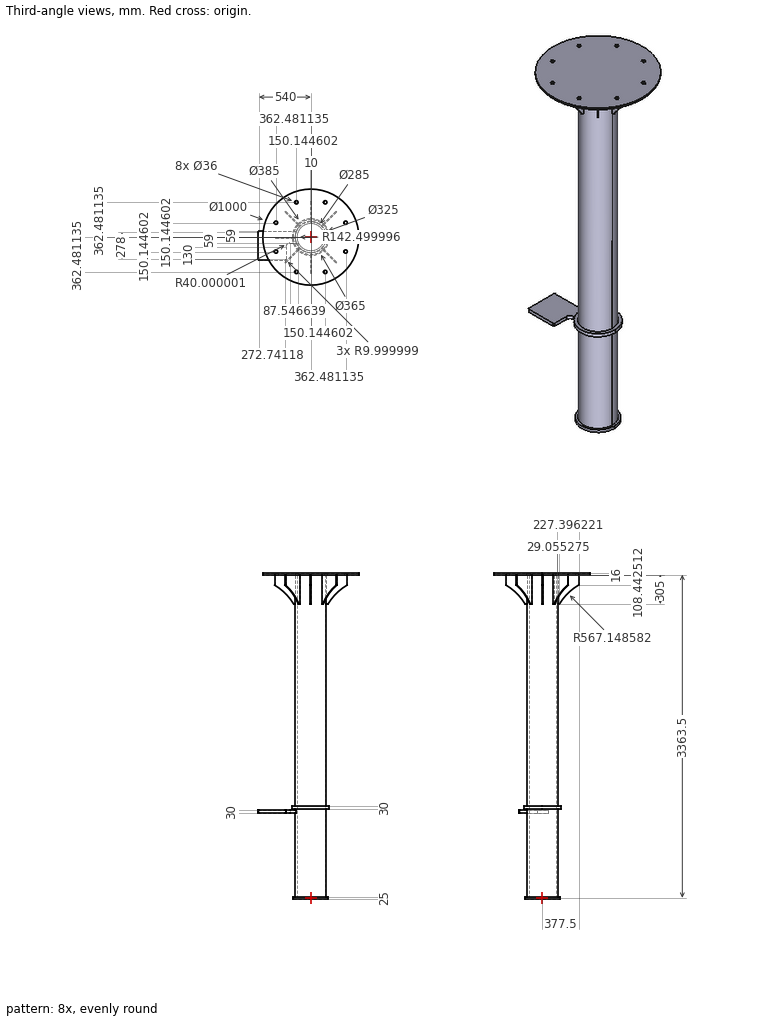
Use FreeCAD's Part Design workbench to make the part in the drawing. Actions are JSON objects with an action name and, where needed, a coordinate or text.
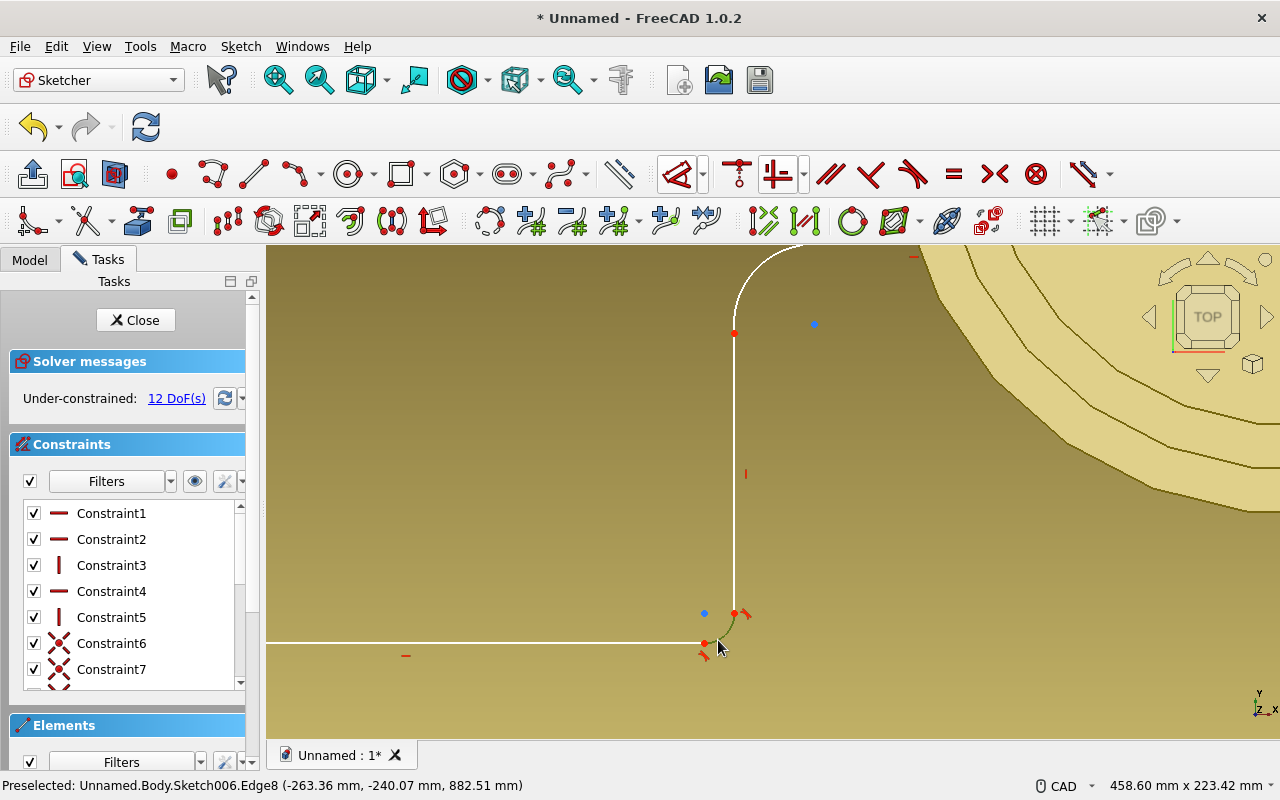
{"action": "scroll", "coordinate": [718, 640], "scroll_direction": "down", "scroll_amount": 4}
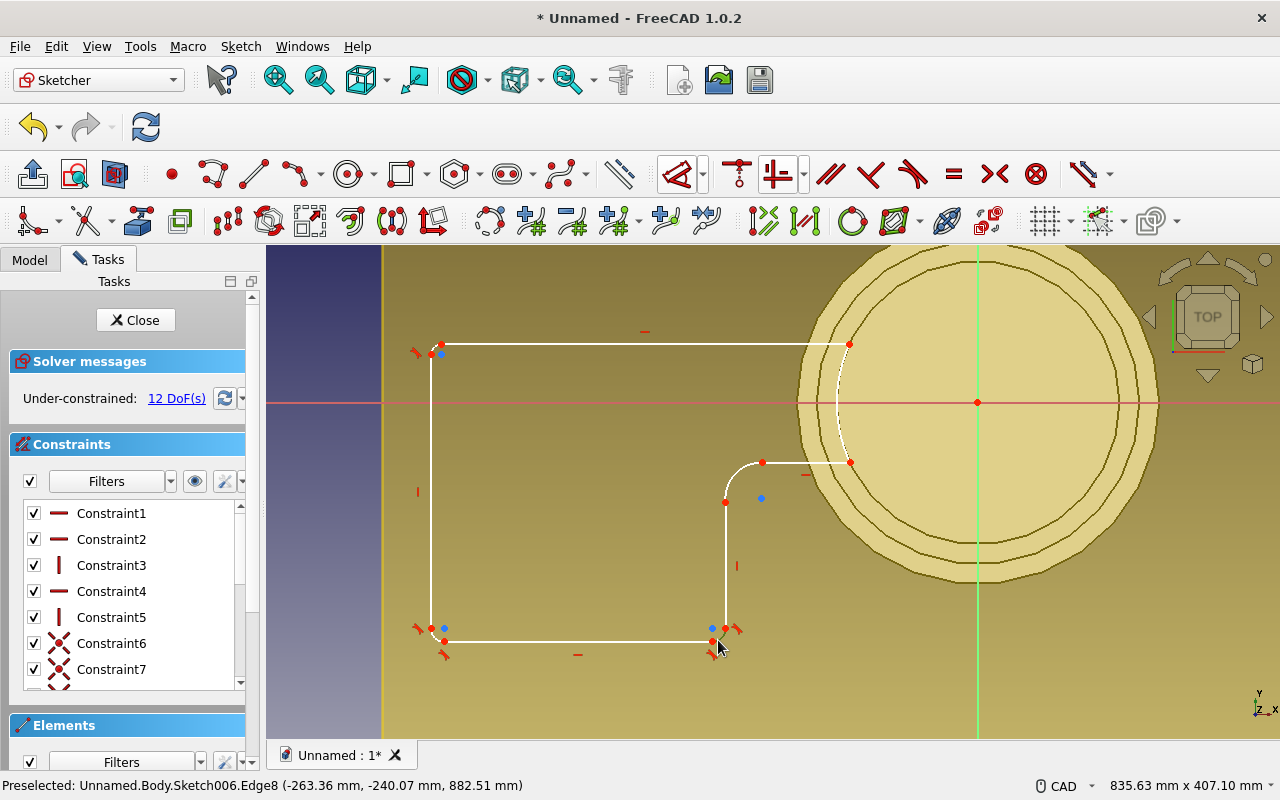
{"action": "scroll", "coordinate": [433, 635], "scroll_direction": "up", "scroll_amount": 5}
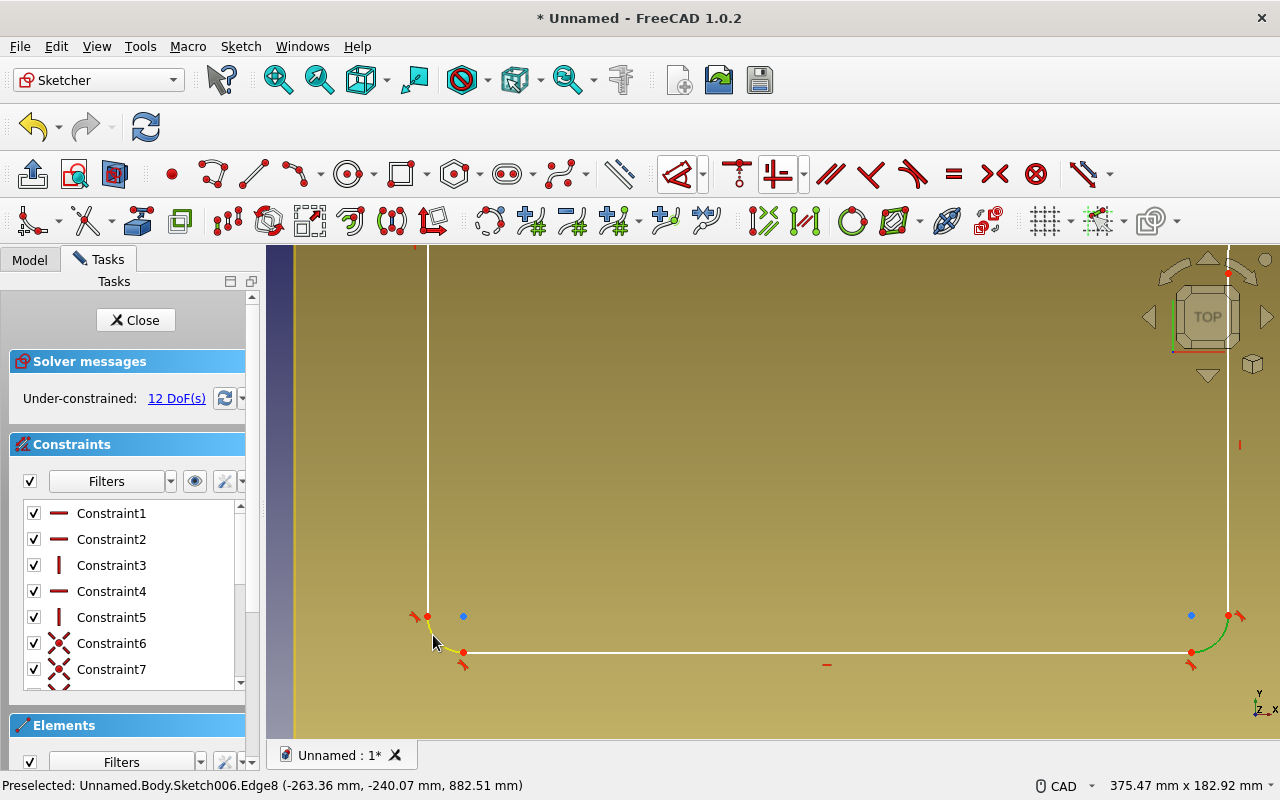
{"action": "left_click", "coordinate": [432, 633]}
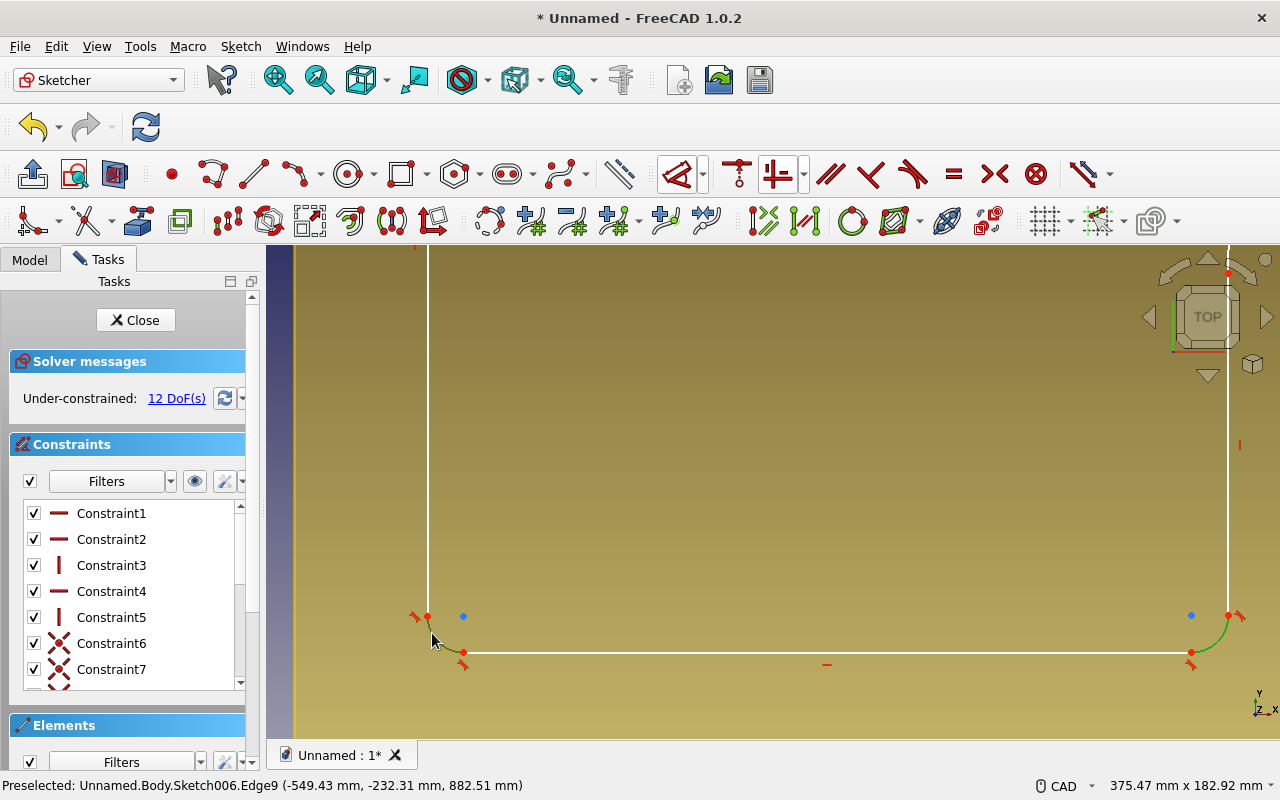
{"action": "scroll", "coordinate": [433, 635], "scroll_direction": "down", "scroll_amount": 5}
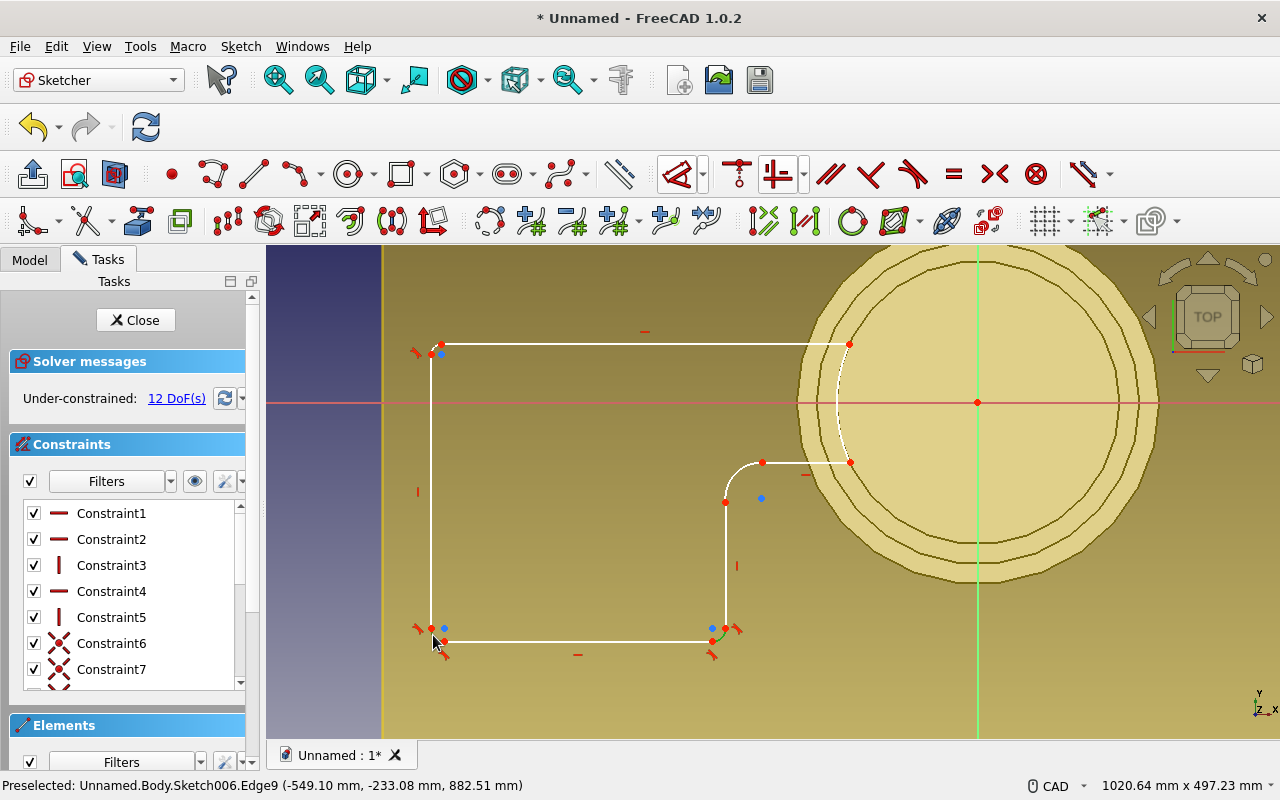
{"action": "scroll", "coordinate": [437, 345], "scroll_direction": "up", "scroll_amount": 6}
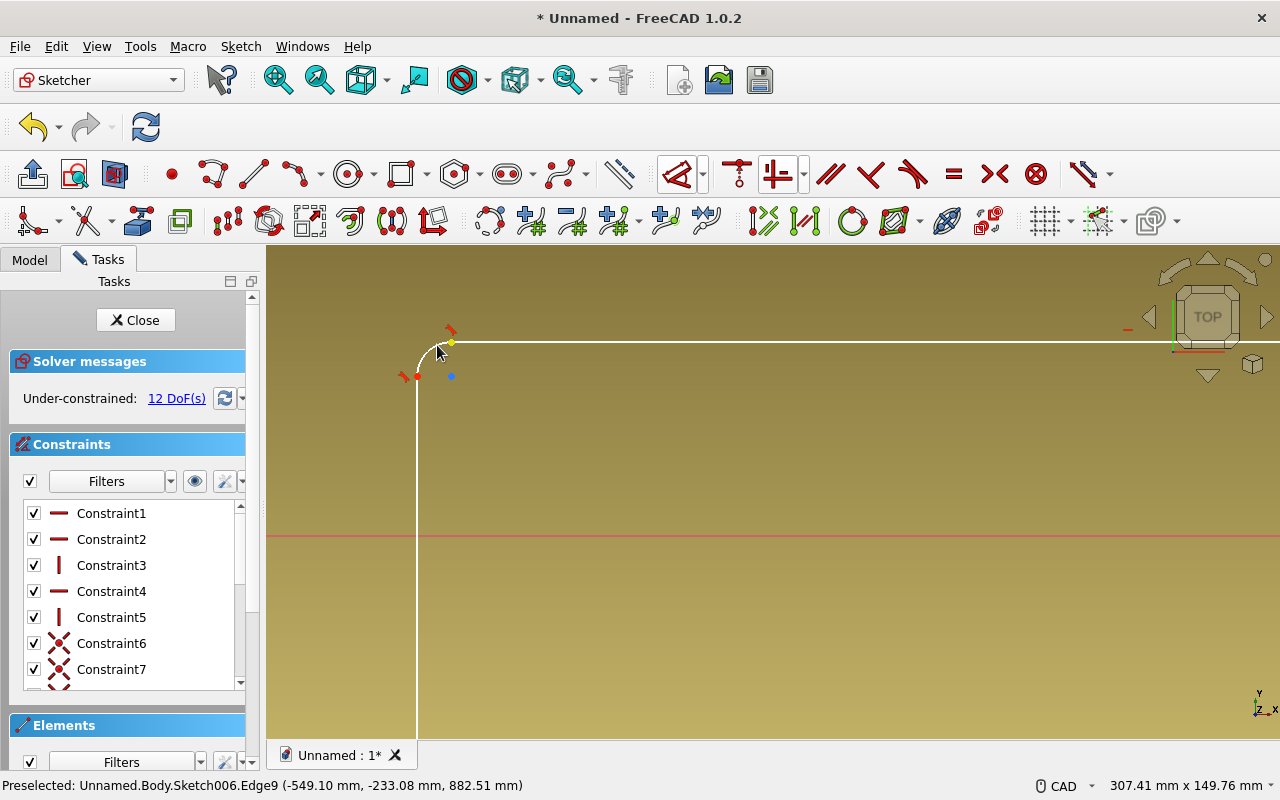
{"action": "left_click", "coordinate": [436, 346]}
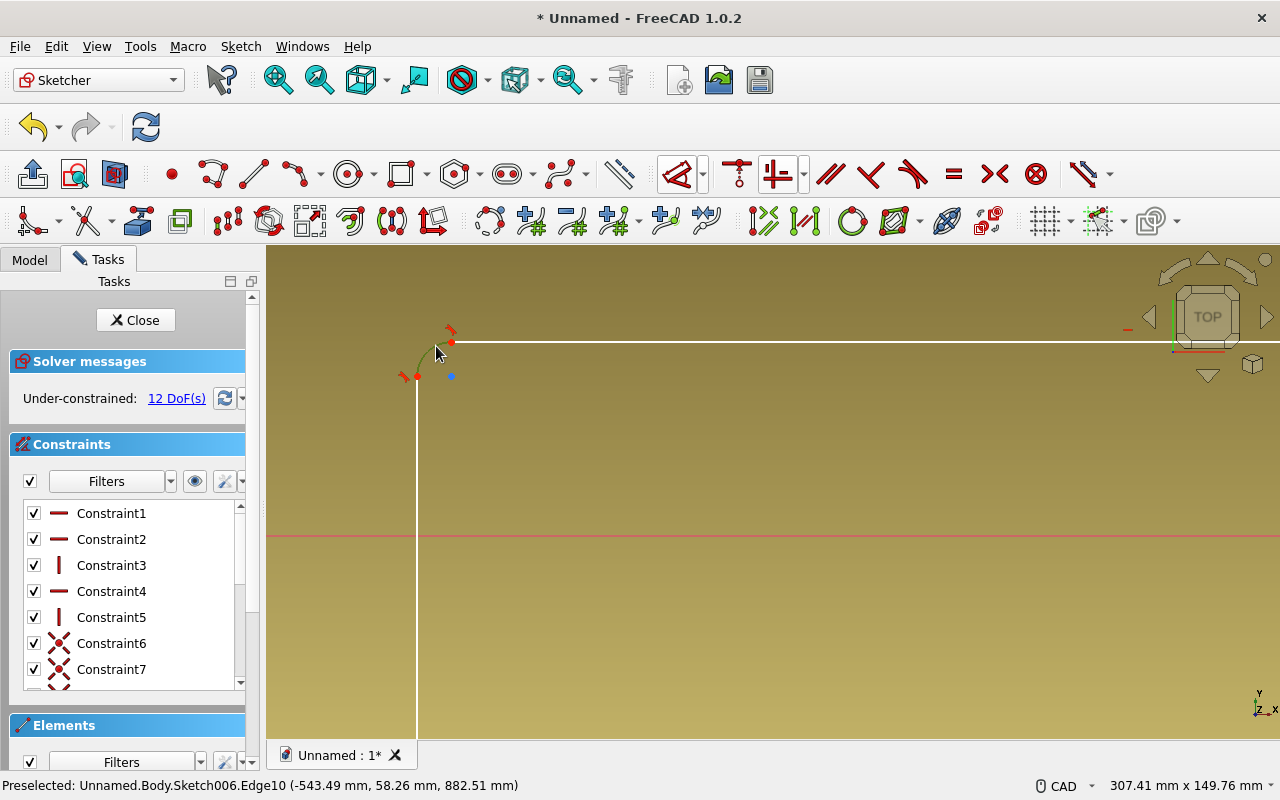
{"action": "key", "text": "e"}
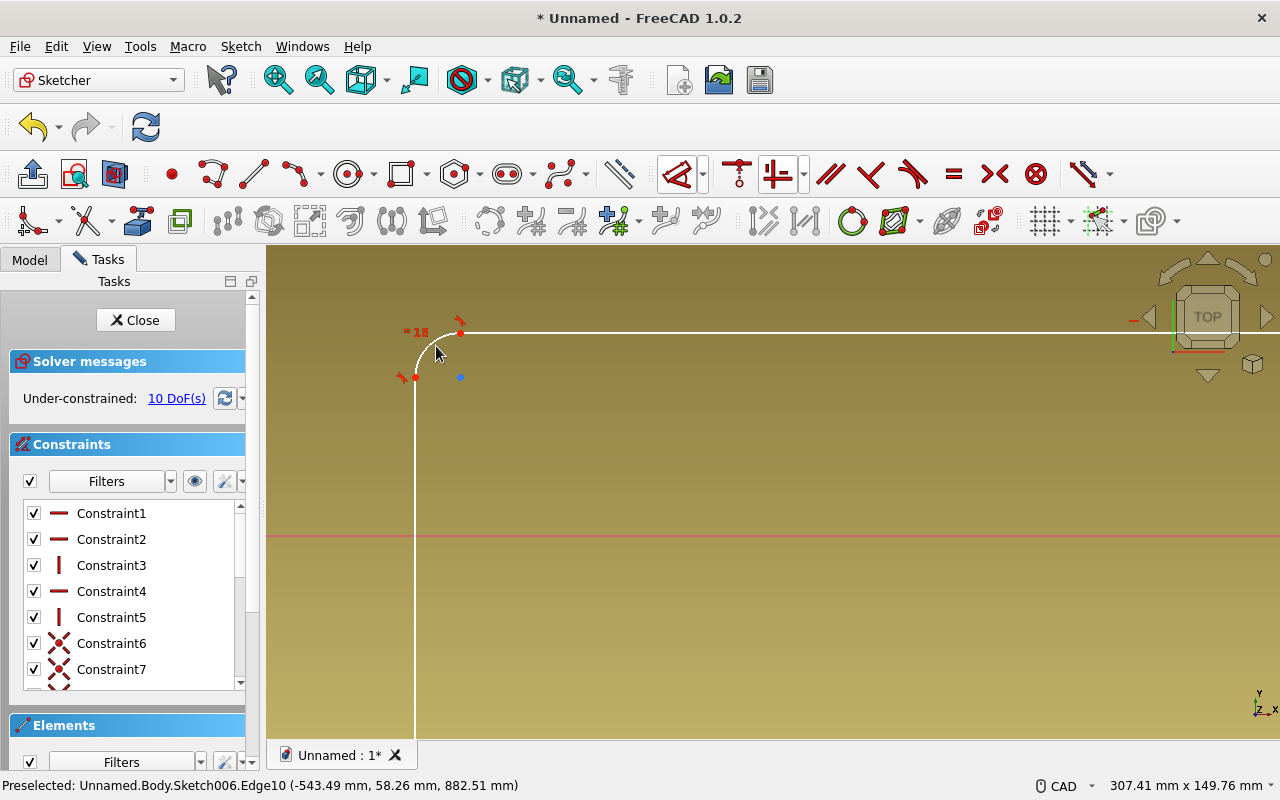
{"action": "scroll", "coordinate": [437, 345], "scroll_direction": "down", "scroll_amount": 6}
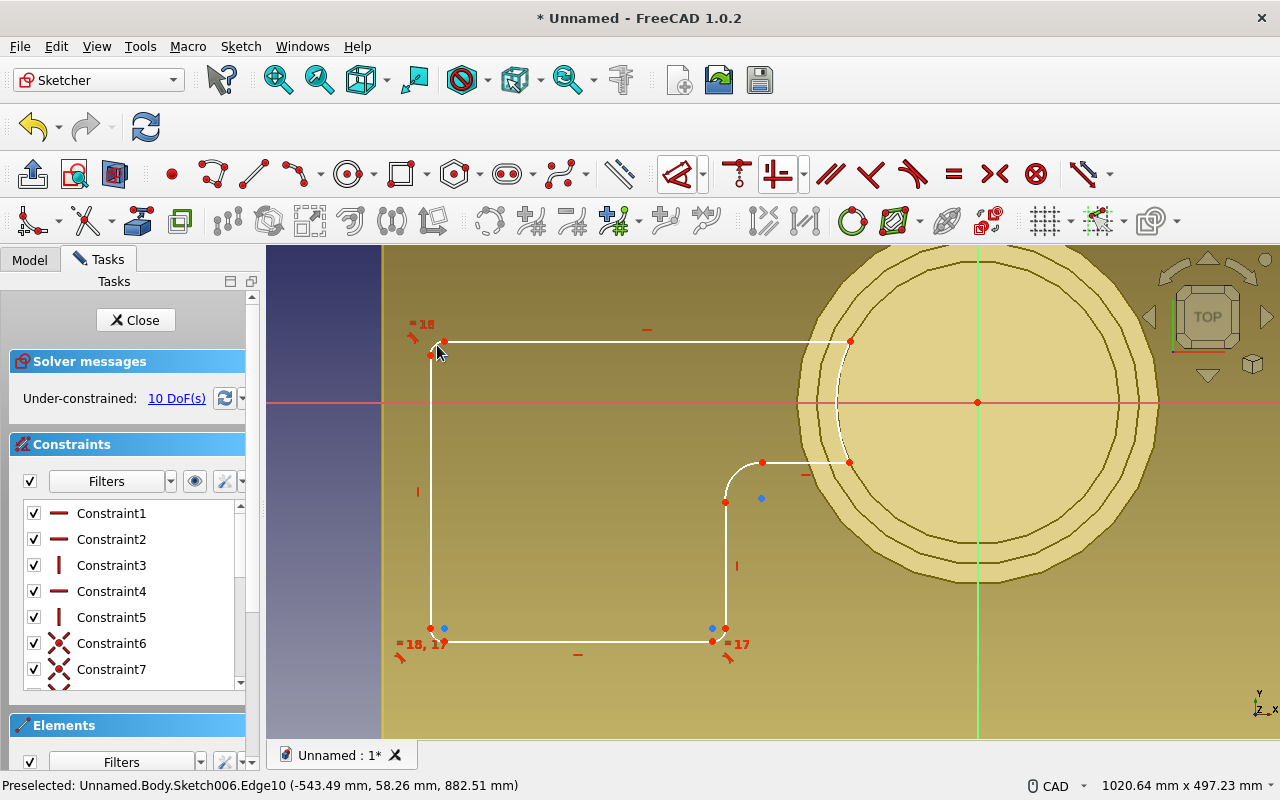
{"action": "left_click", "coordinate": [839, 377]}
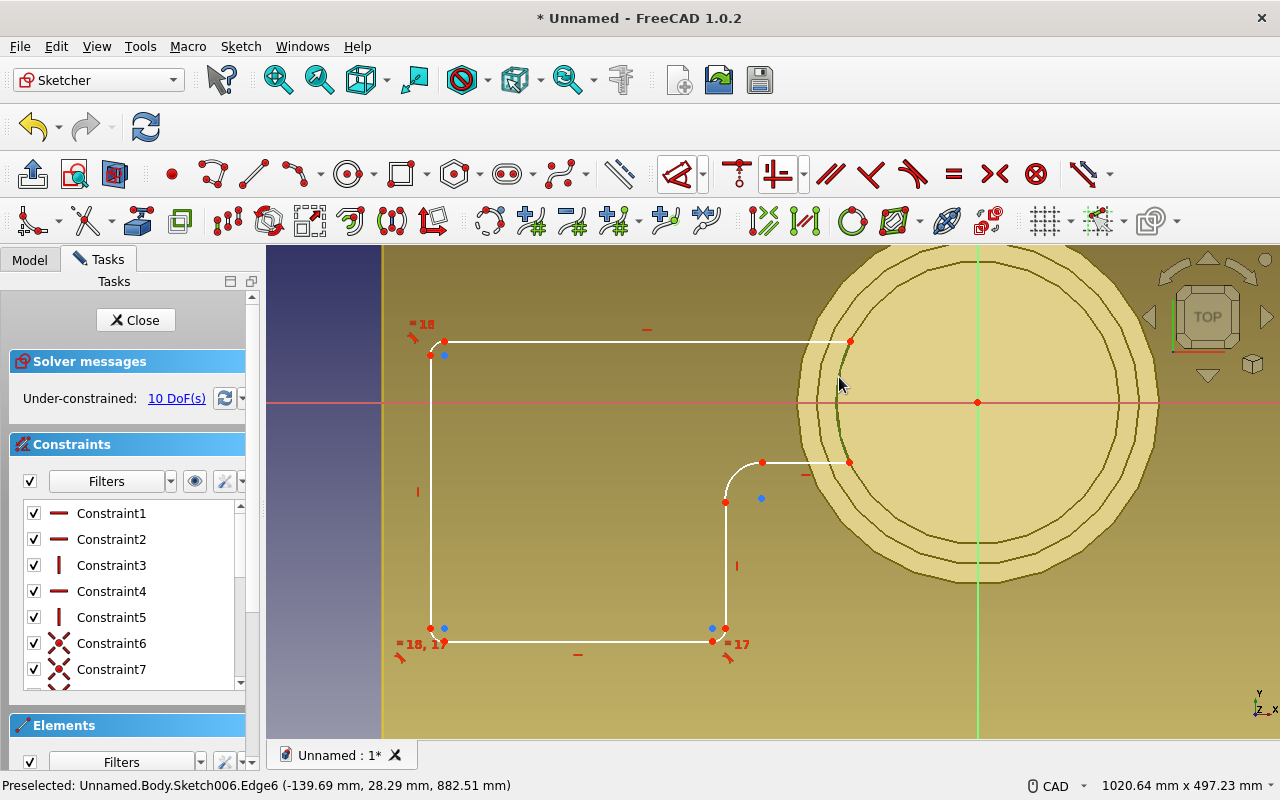
{"action": "key", "text": "k r"}